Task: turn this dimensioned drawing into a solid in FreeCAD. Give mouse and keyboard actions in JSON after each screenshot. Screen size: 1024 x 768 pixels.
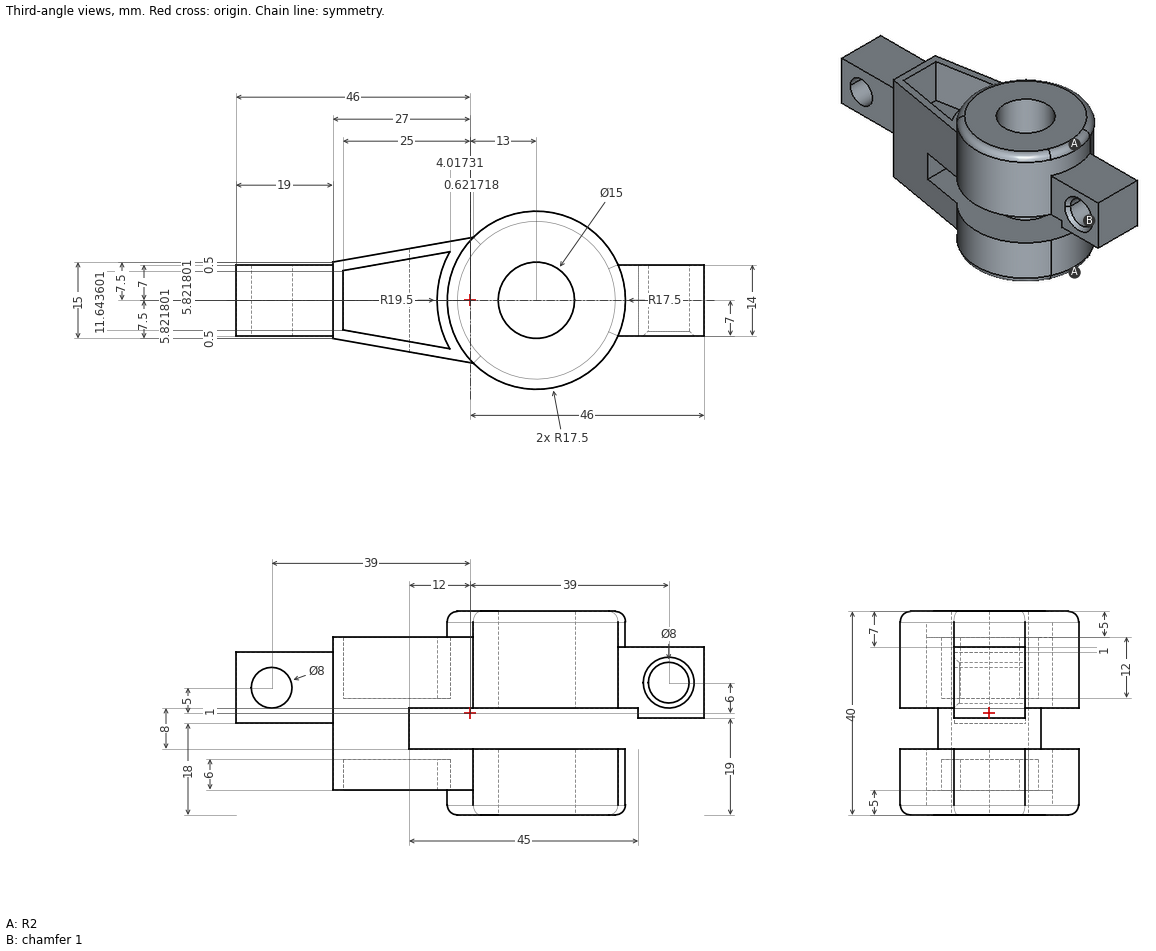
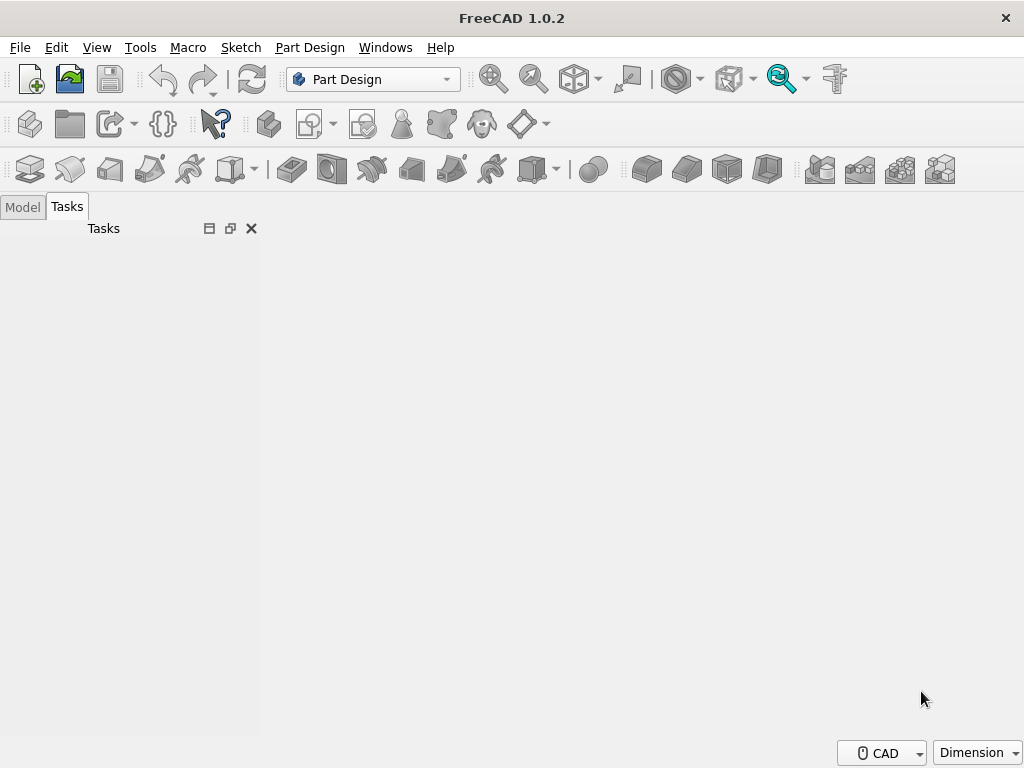
{"action": "left_click", "coordinate": [30, 80]}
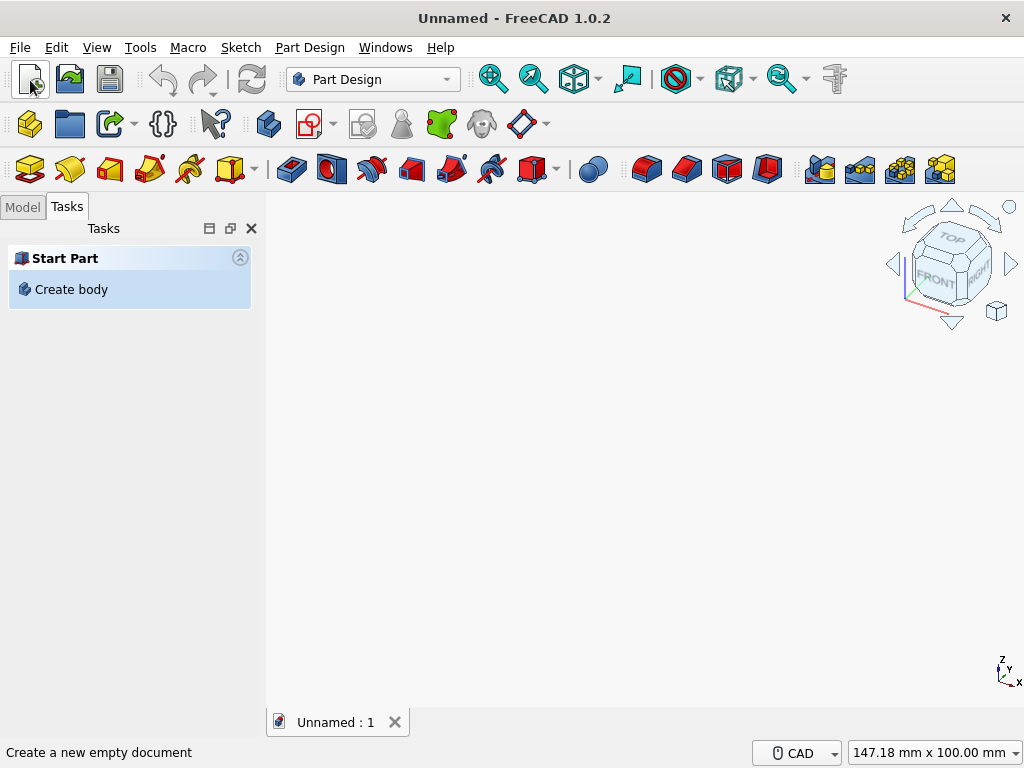
{"action": "left_click", "coordinate": [310, 124]}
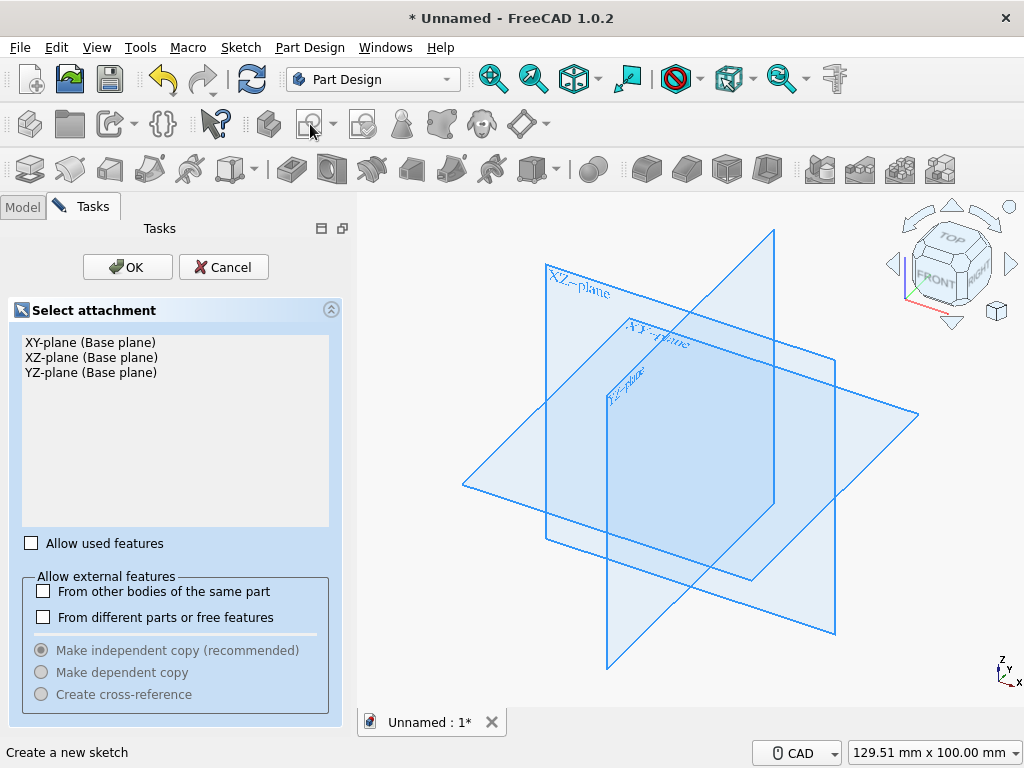
{"action": "left_click", "coordinate": [82, 342]}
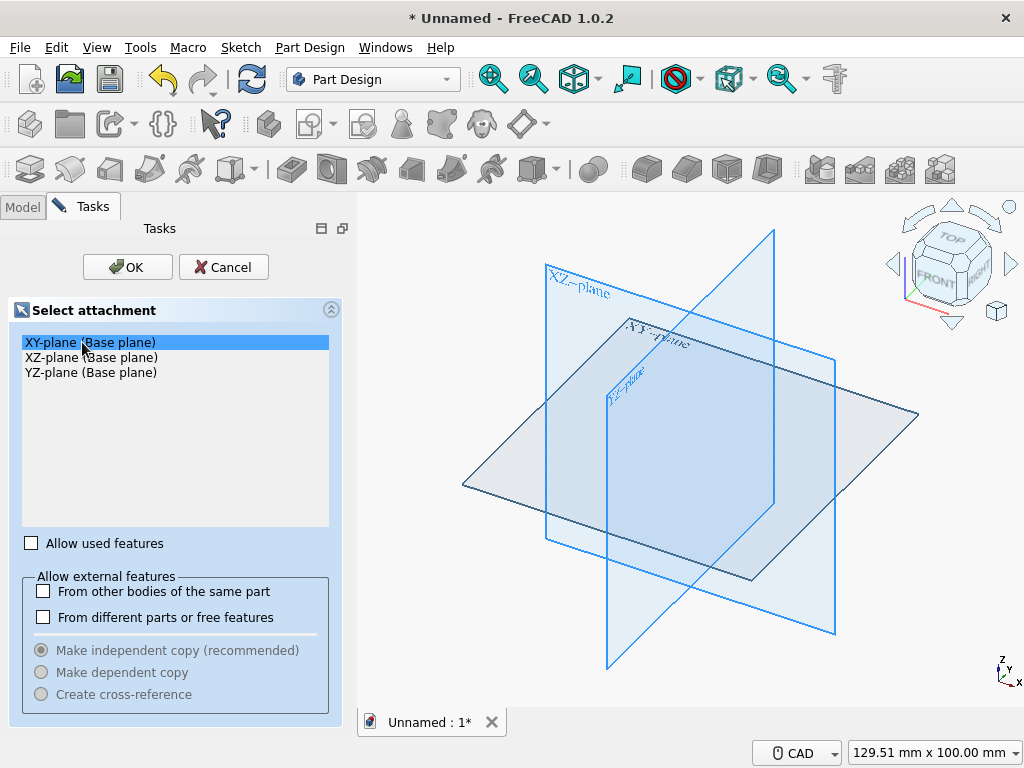
{"action": "left_click", "coordinate": [128, 267]}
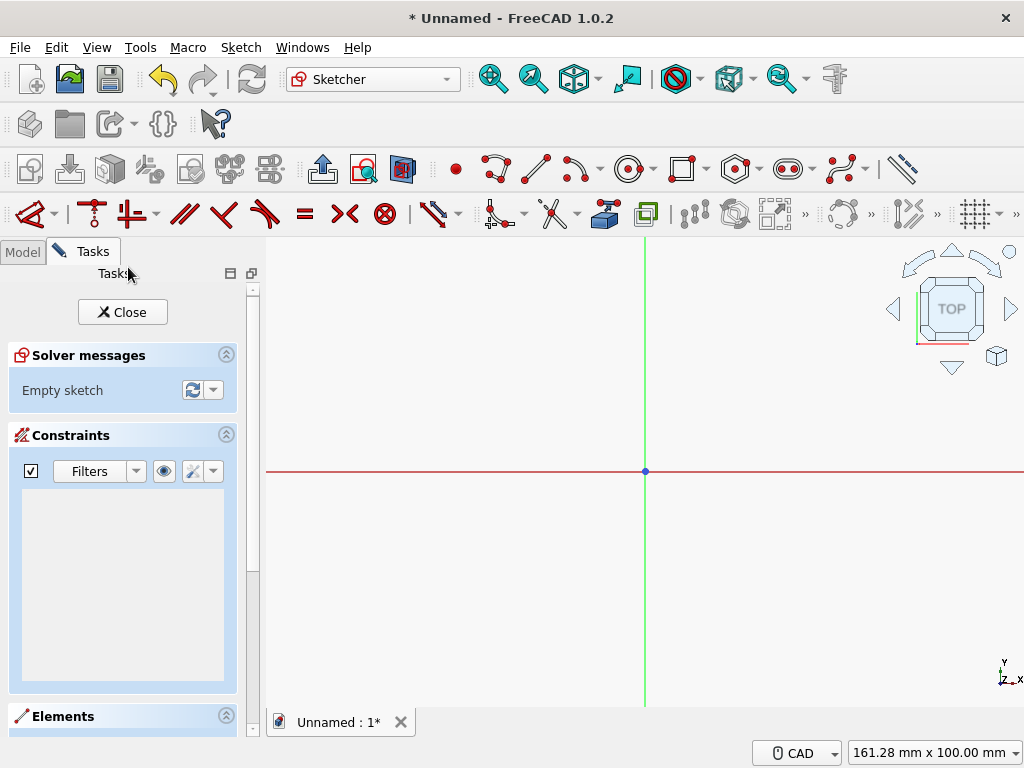
{"action": "scroll", "coordinate": [294, 472], "scroll_direction": "down", "scroll_amount": 1}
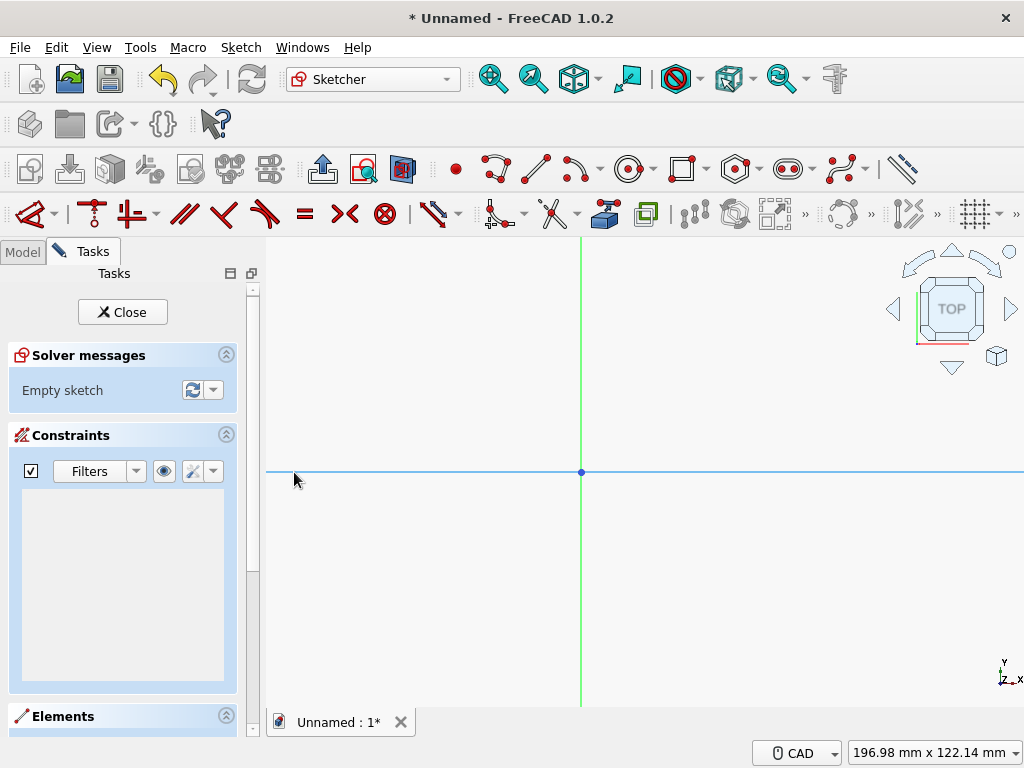
{"action": "left_click", "coordinate": [496, 170]}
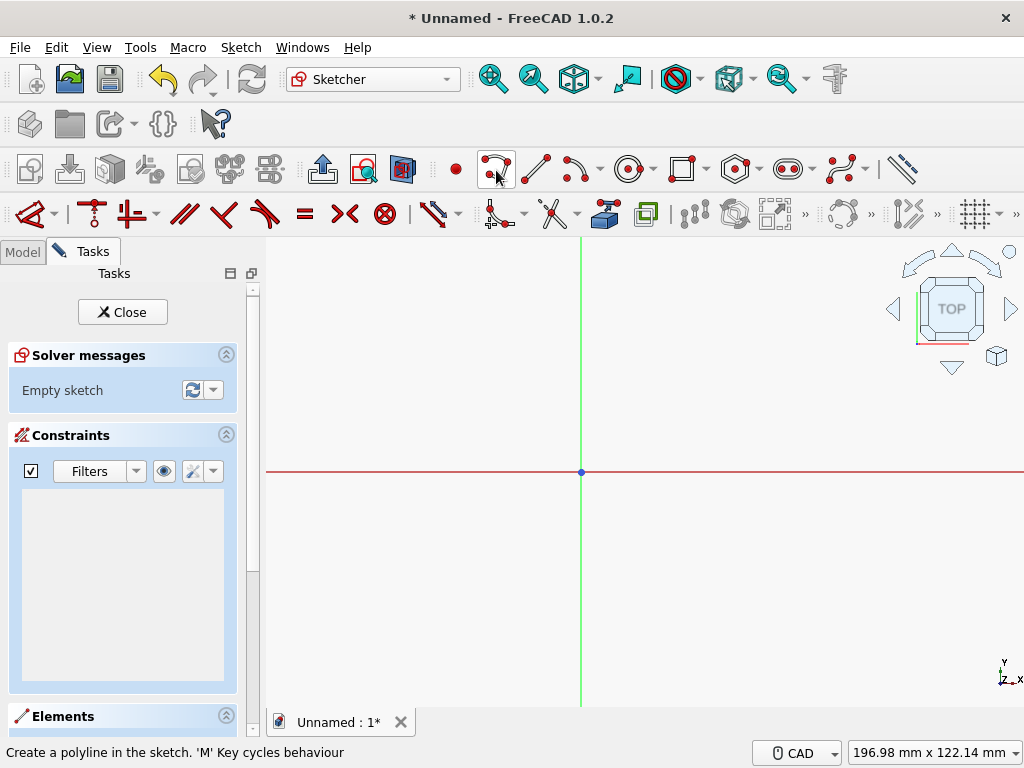
{"action": "left_click", "coordinate": [693, 499]}
{"action": "left_click", "coordinate": [758, 499]}
{"action": "left_click", "coordinate": [758, 445]}
{"action": "left_click", "coordinate": [693, 445]}
{"action": "right_click", "coordinate": [693, 445]}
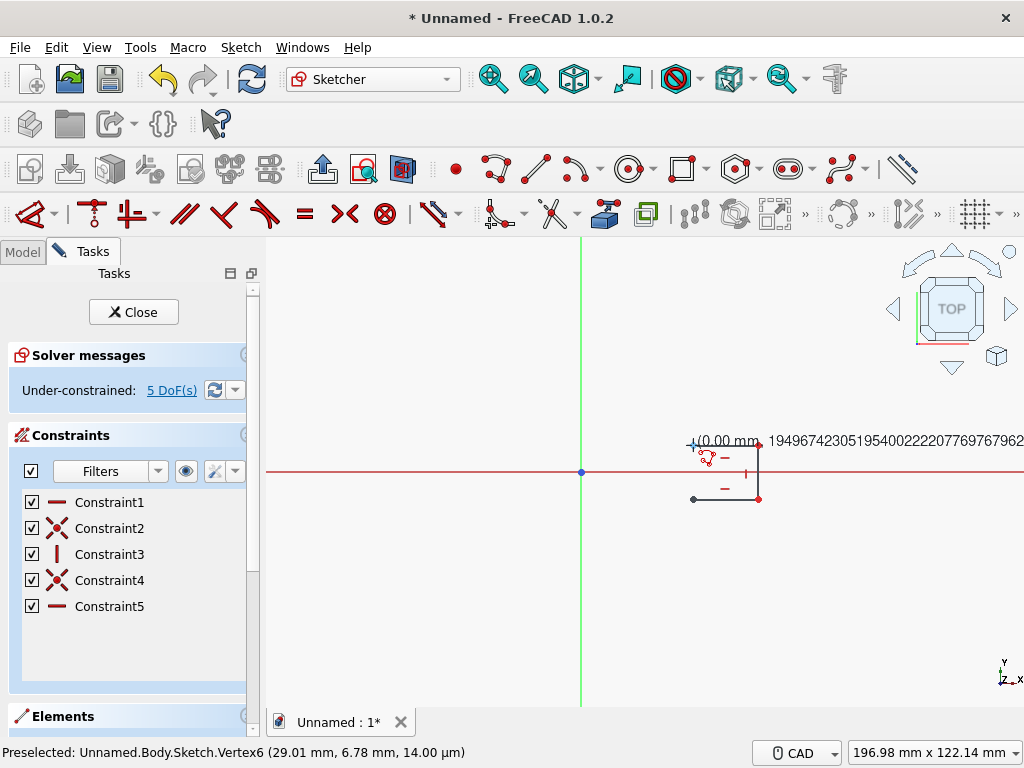
{"action": "scroll", "coordinate": [584, 424], "scroll_direction": "up", "scroll_amount": 10}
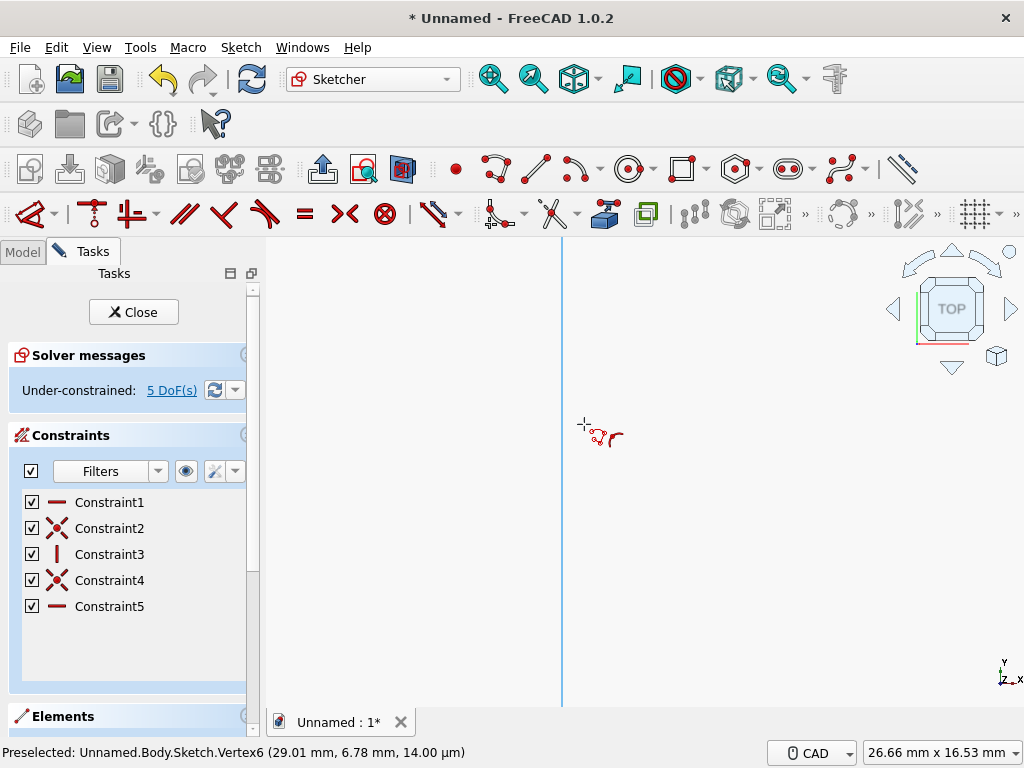
{"action": "left_click", "coordinate": [580, 425]}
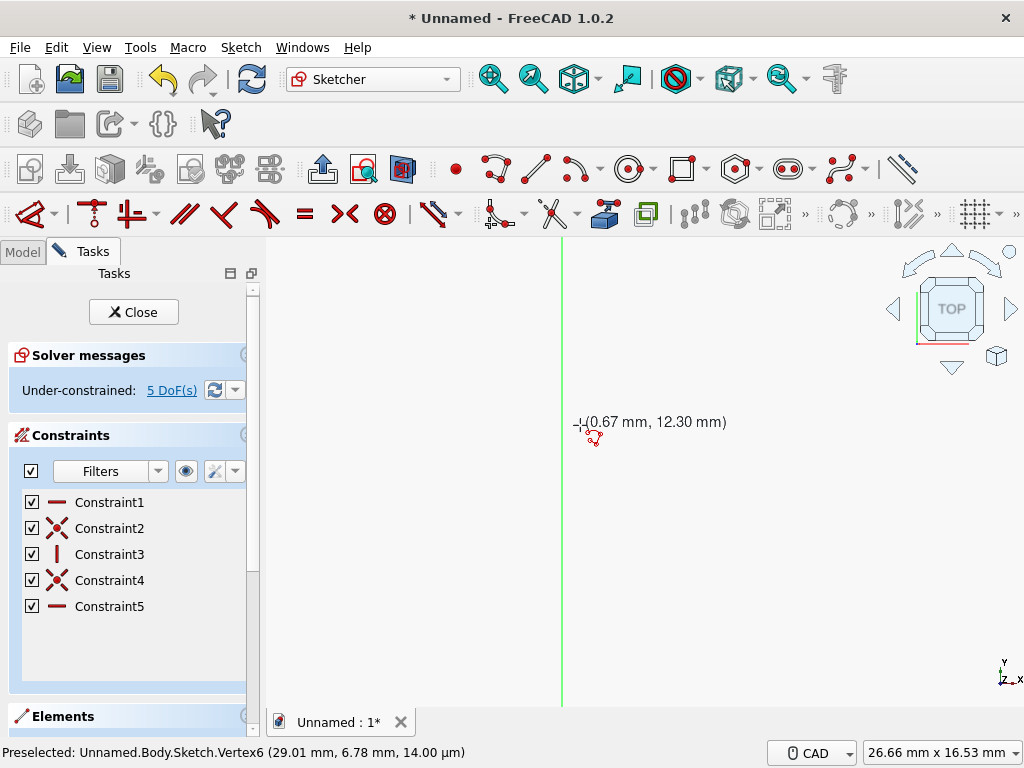
{"action": "scroll", "coordinate": [579, 412], "scroll_direction": "down", "scroll_amount": 9}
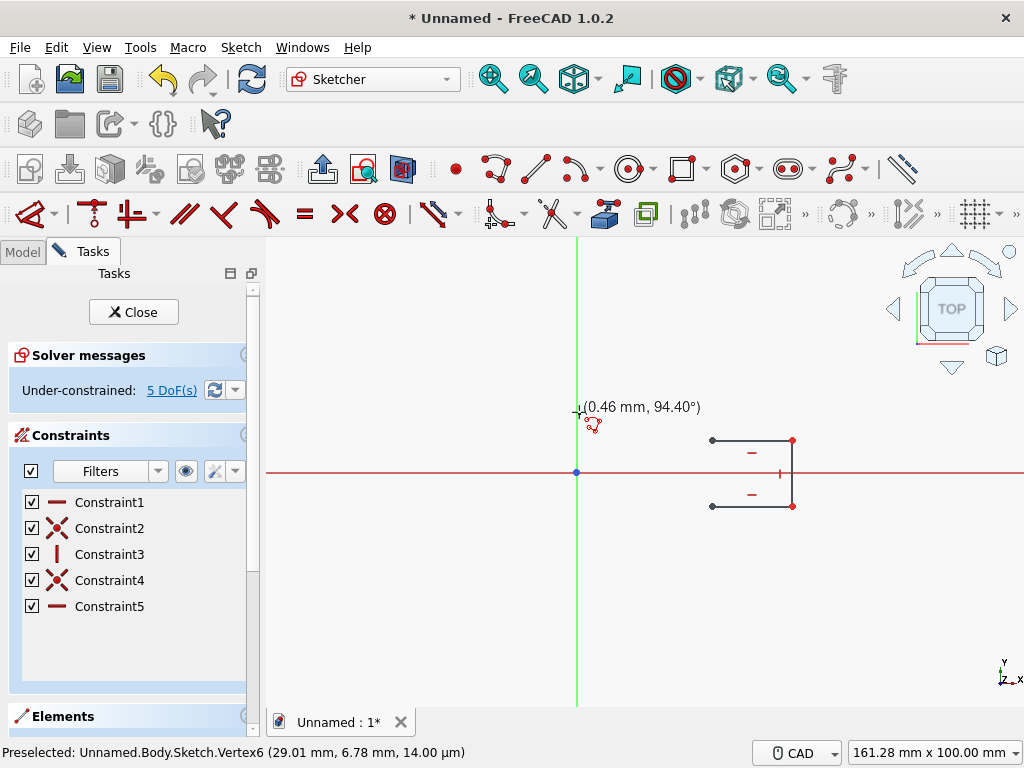
{"action": "left_click", "coordinate": [450, 437]}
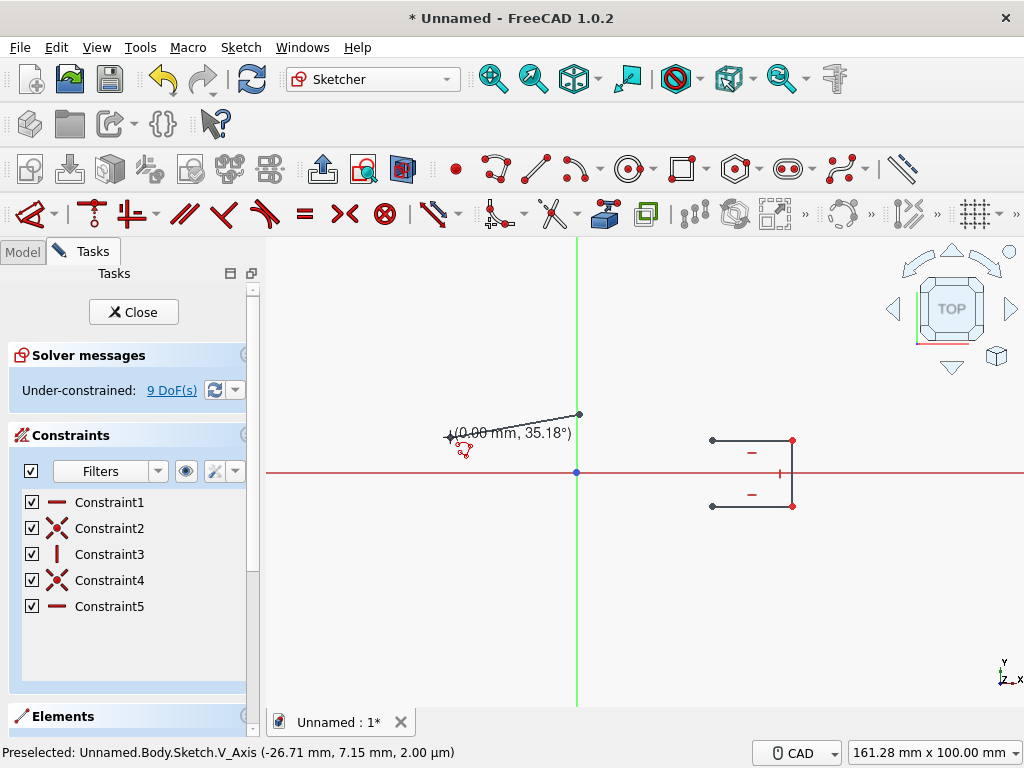
{"action": "scroll", "coordinate": [450, 440], "scroll_direction": "up", "scroll_amount": 10}